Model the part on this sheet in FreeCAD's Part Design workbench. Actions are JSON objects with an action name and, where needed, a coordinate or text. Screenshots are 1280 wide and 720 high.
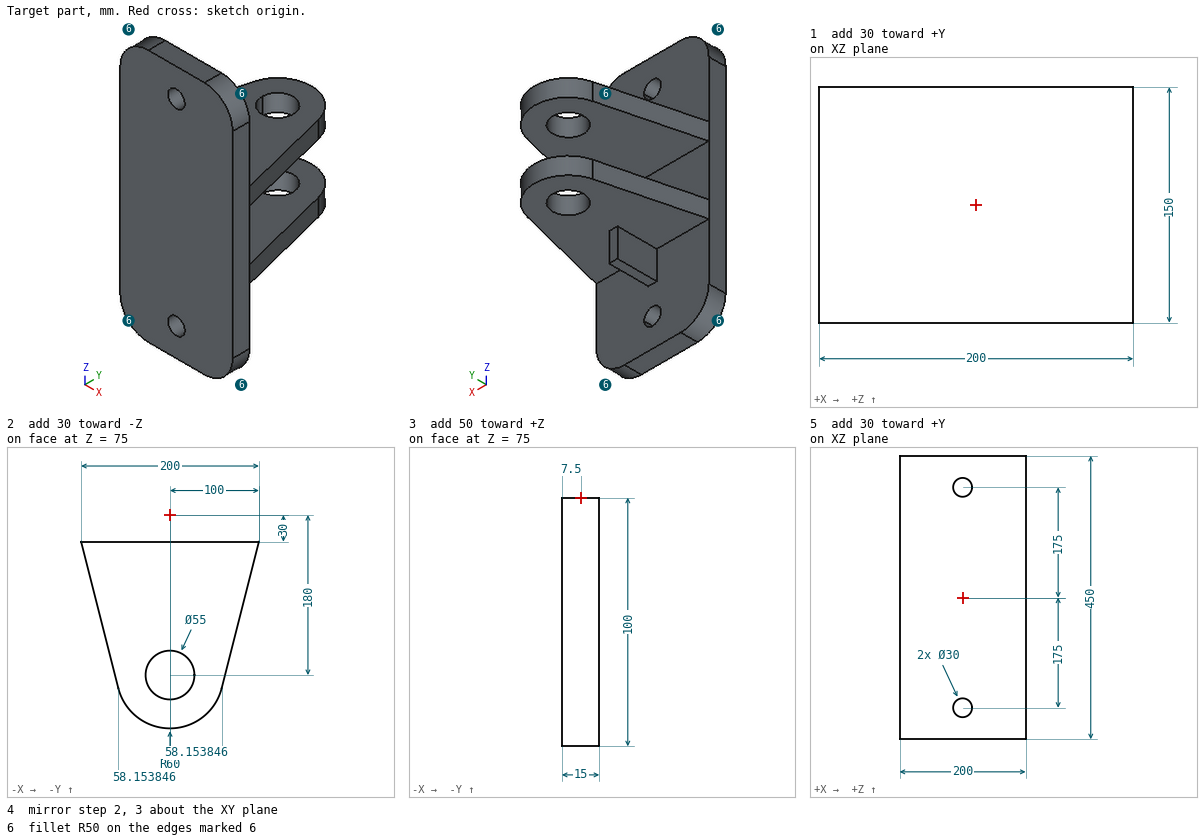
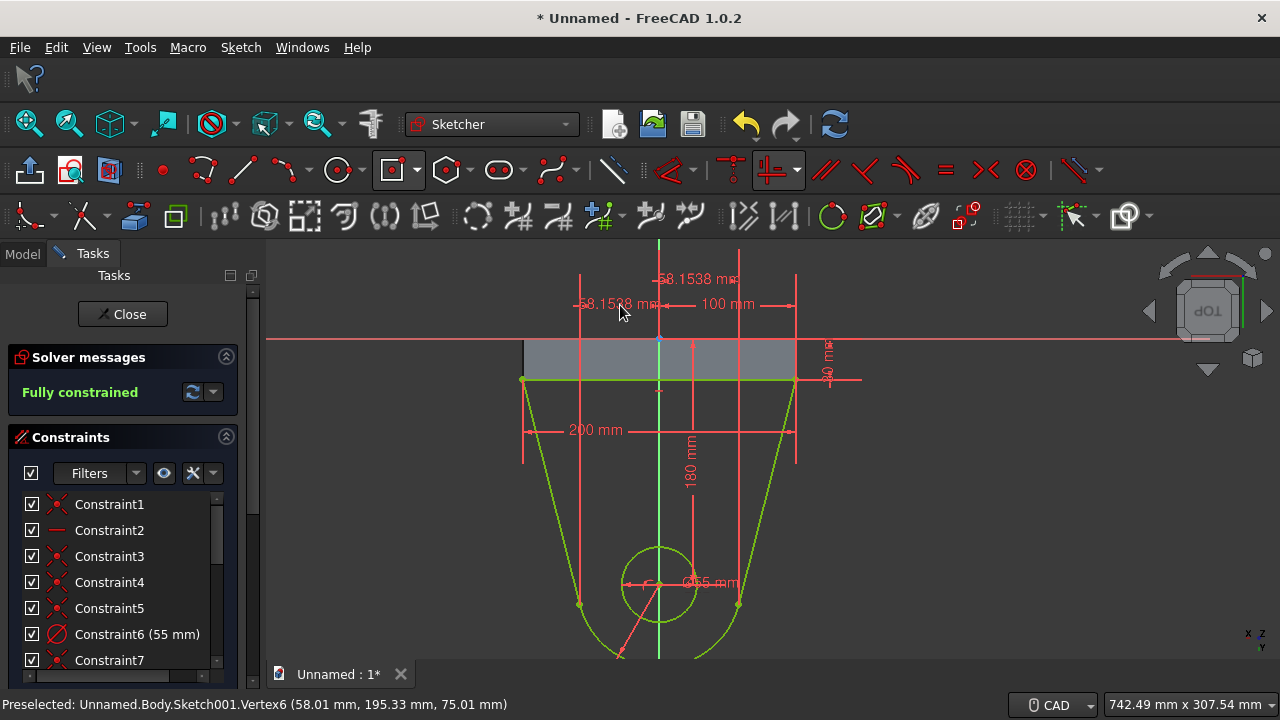
{"action": "left_click", "coordinate": [123, 314]}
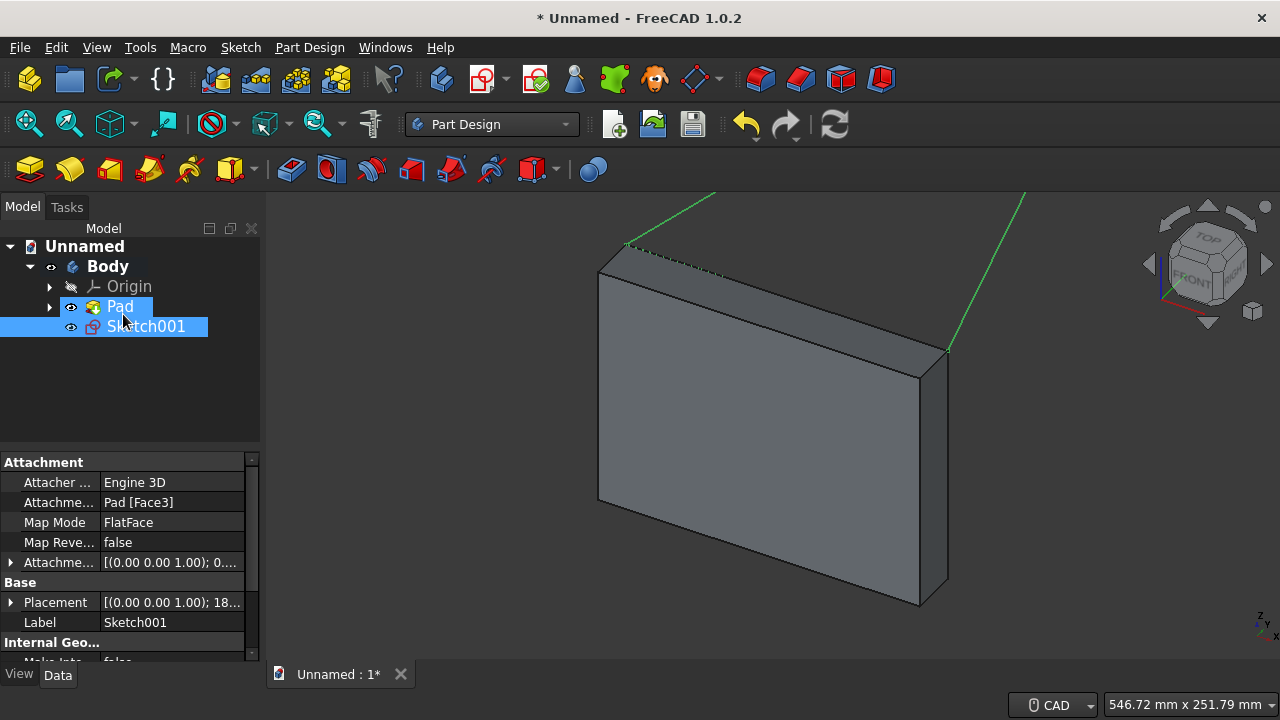
{"action": "left_click", "coordinate": [30, 170]}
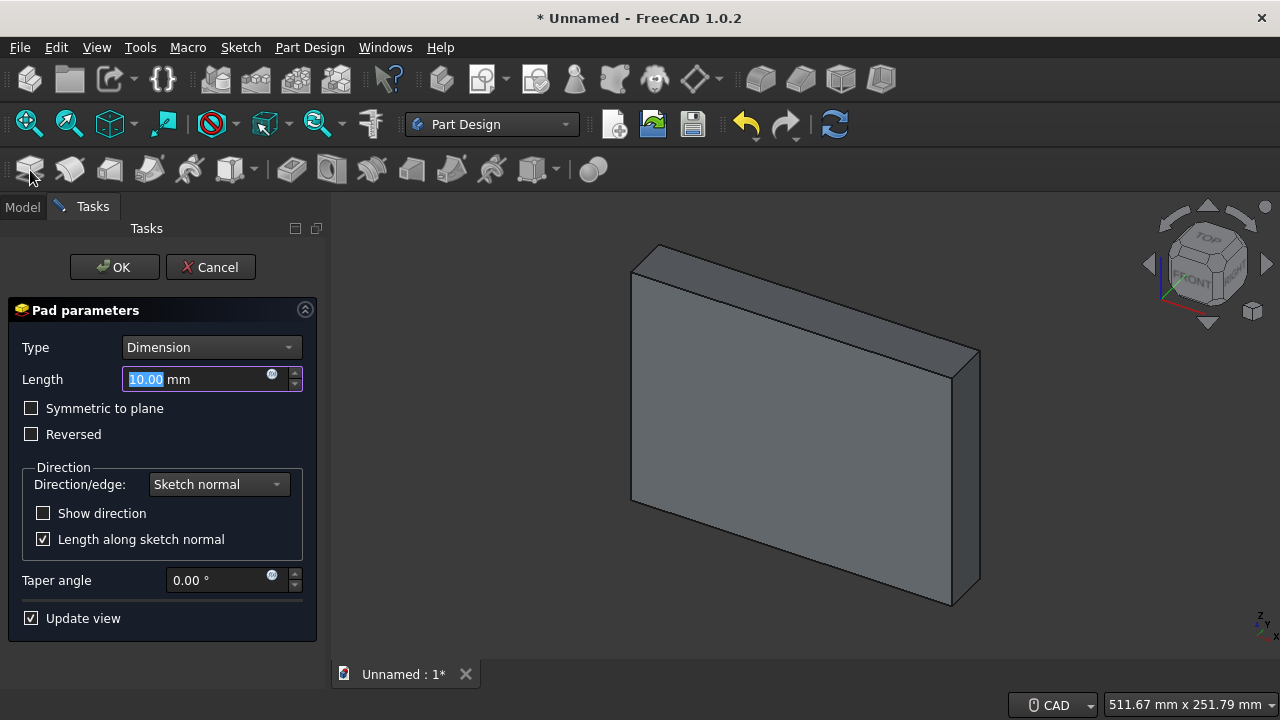
{"action": "type", "text": "30"}
{"action": "key", "text": "Tab"}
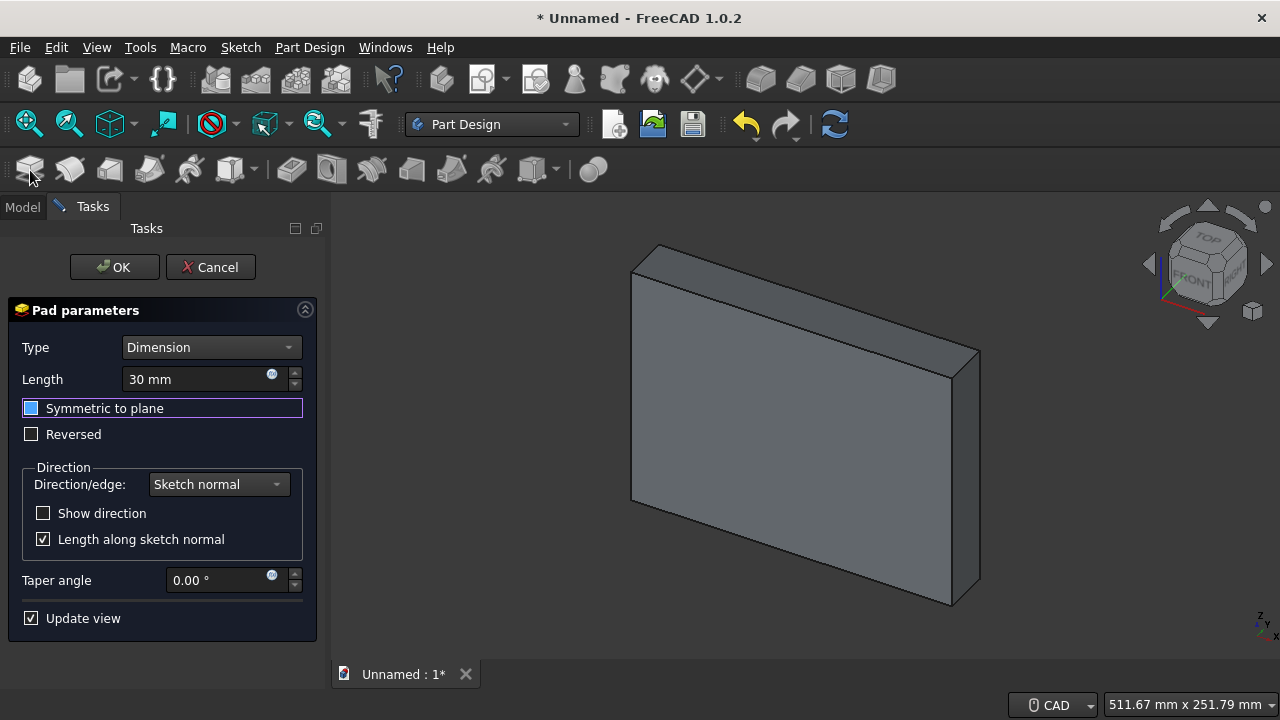
{"action": "left_click", "coordinate": [30, 434]}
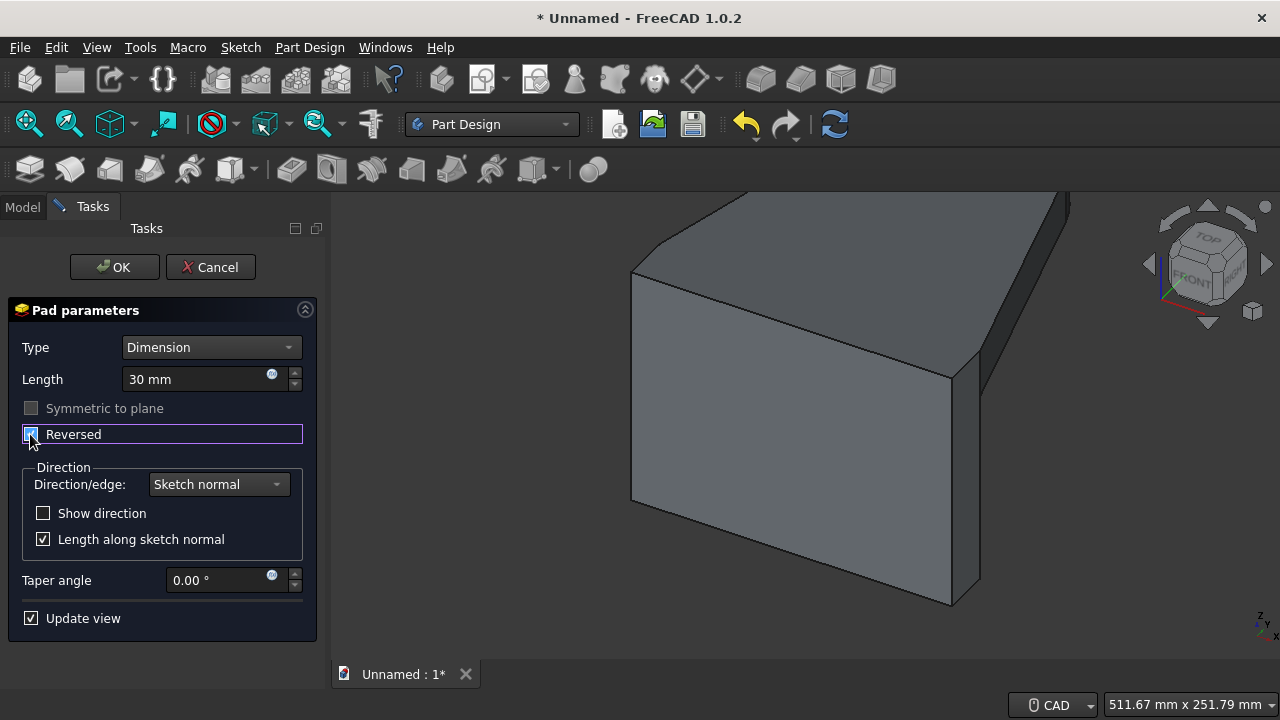
{"action": "left_click", "coordinate": [115, 267]}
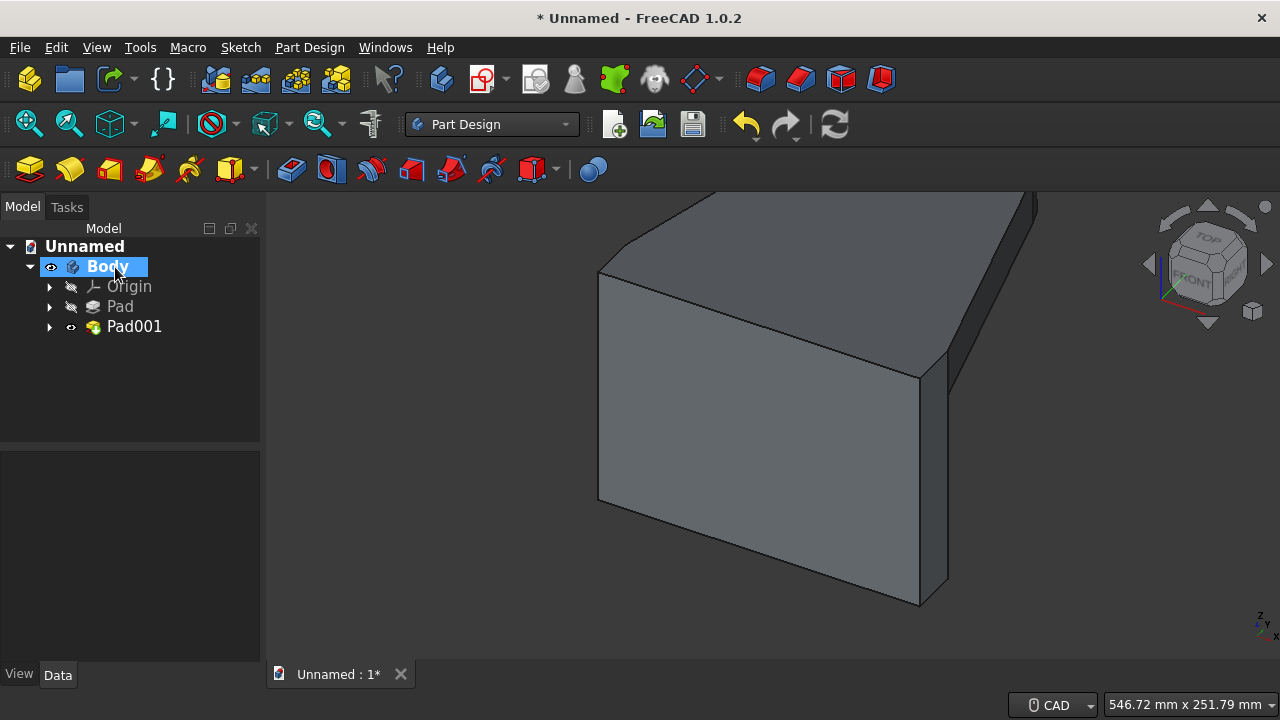
{"action": "key", "text": "v f"}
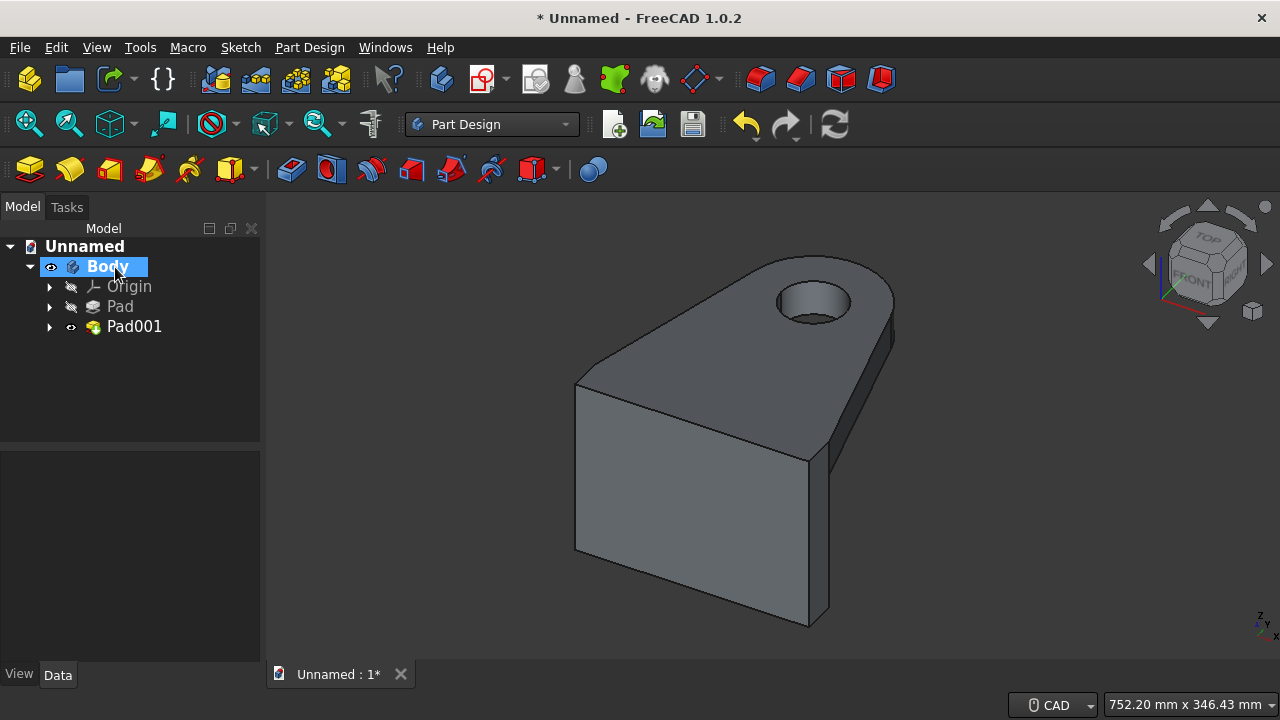
{"action": "left_click", "coordinate": [750, 365]}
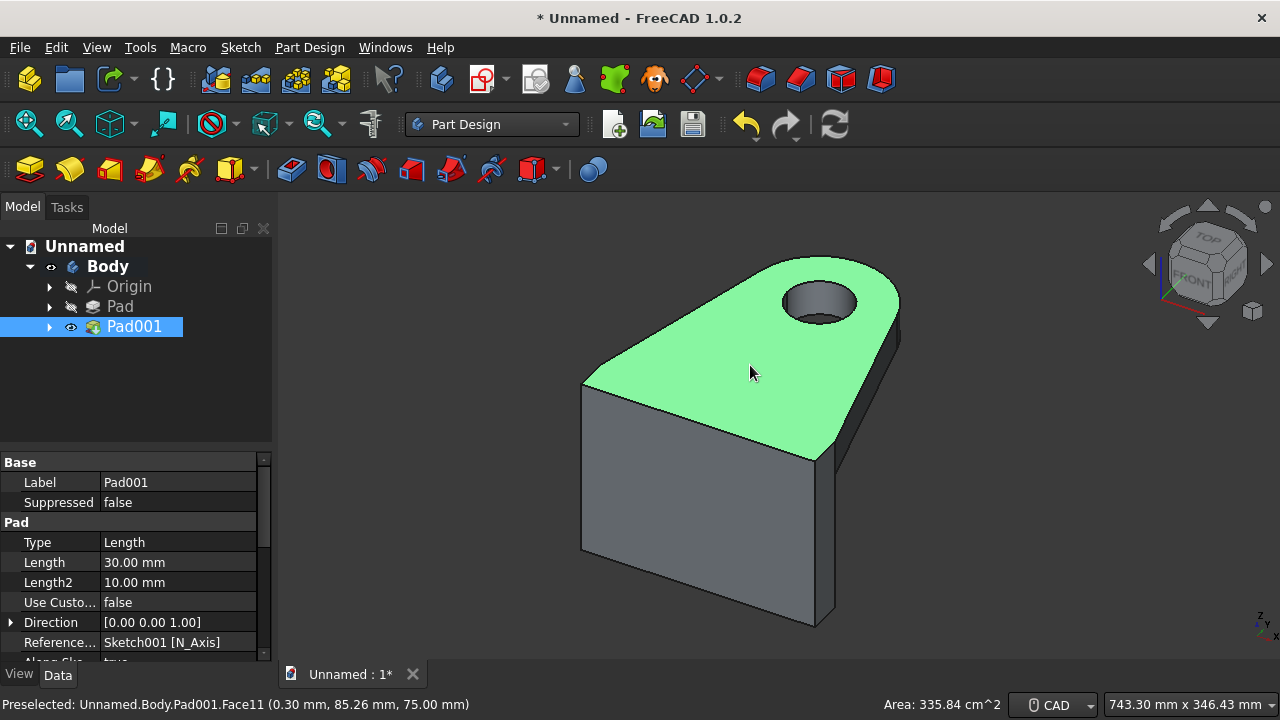
{"action": "left_click", "coordinate": [482, 80]}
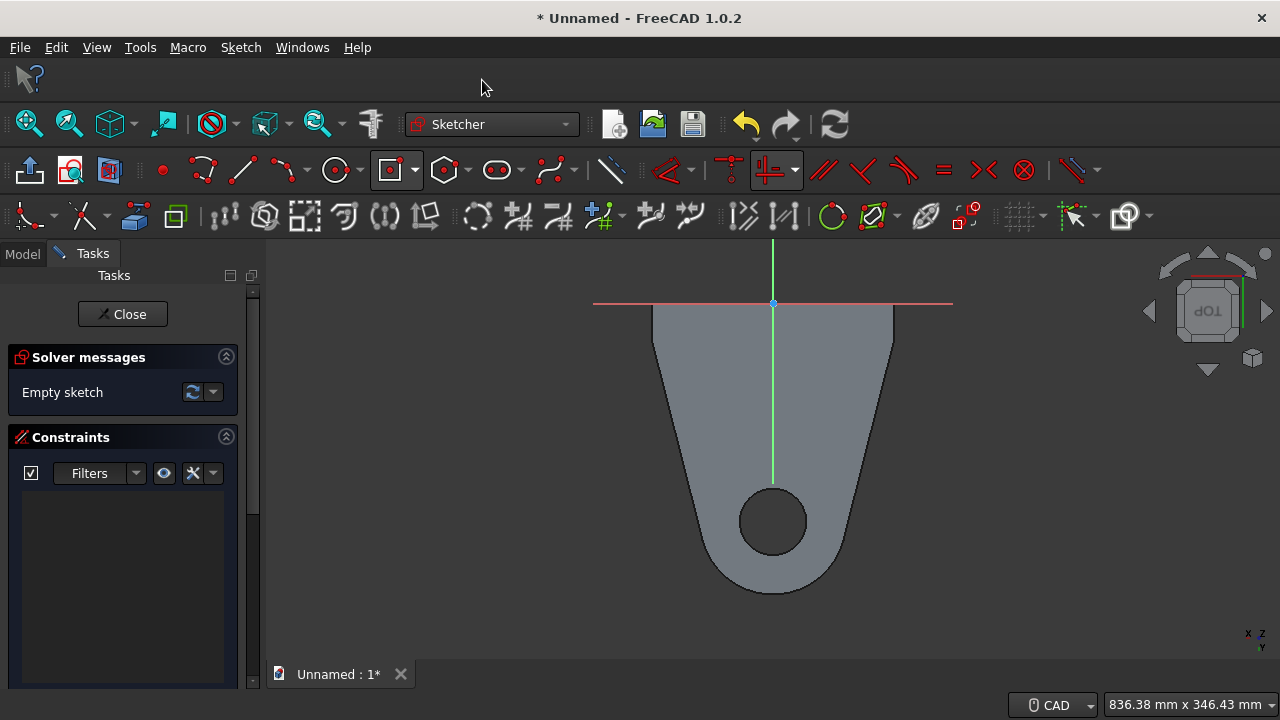
{"action": "scroll", "coordinate": [829, 295], "scroll_direction": "up", "scroll_amount": 4}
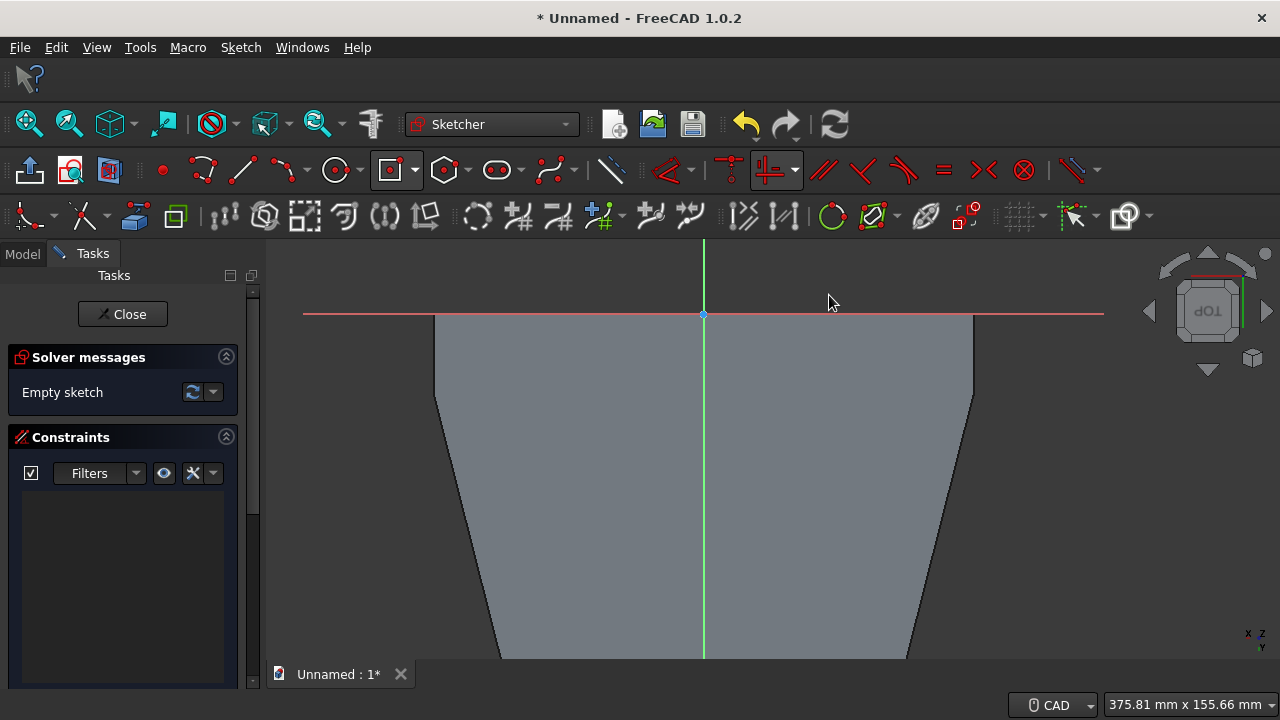
{"action": "key", "text": "g r"}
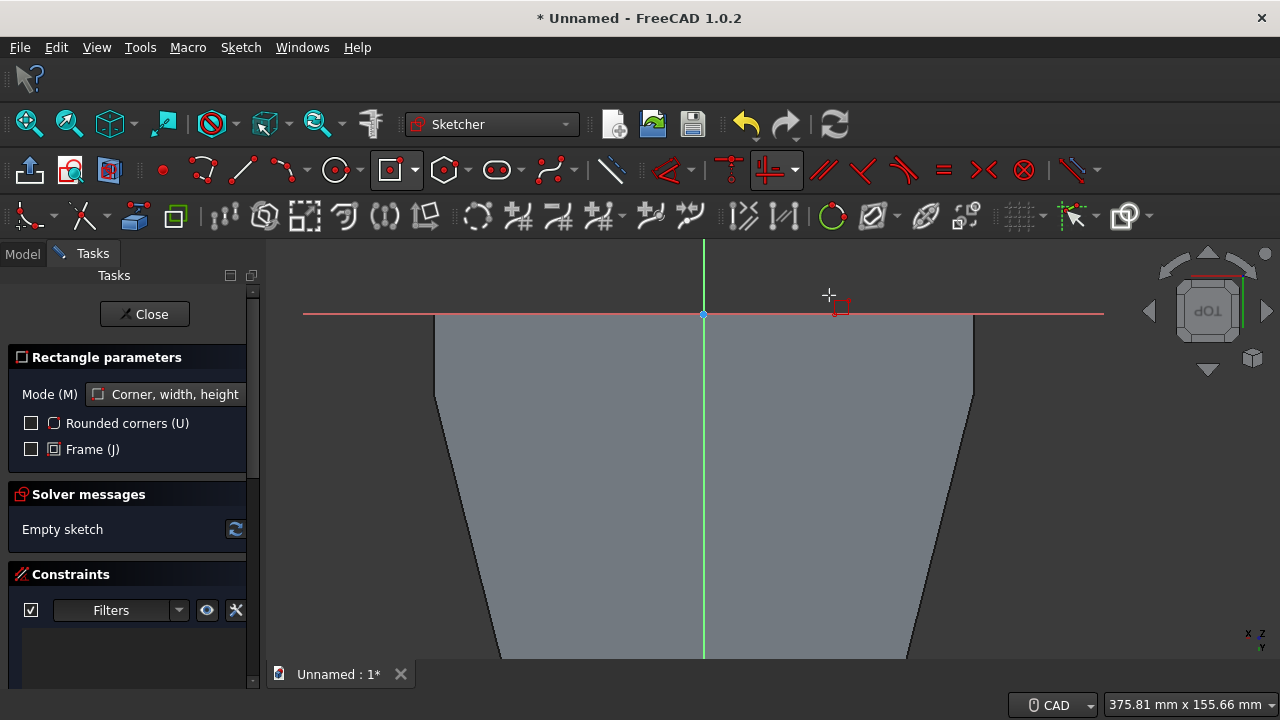
{"action": "left_click", "coordinate": [683, 314]}
{"action": "mouse_move", "coordinate": [724, 584]}